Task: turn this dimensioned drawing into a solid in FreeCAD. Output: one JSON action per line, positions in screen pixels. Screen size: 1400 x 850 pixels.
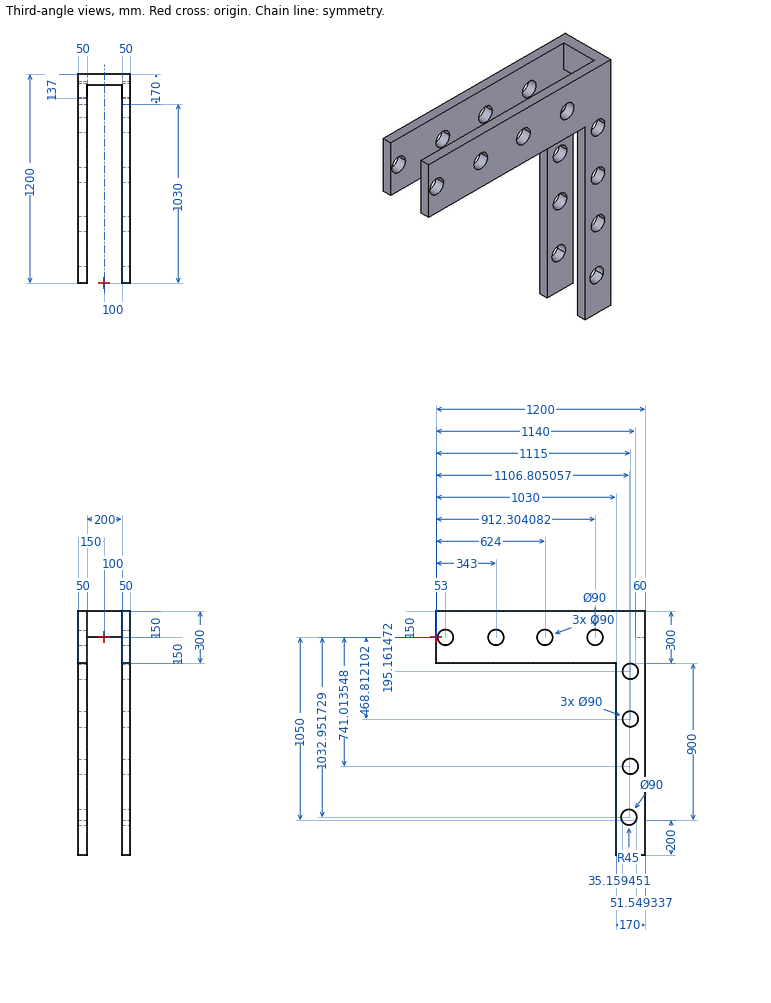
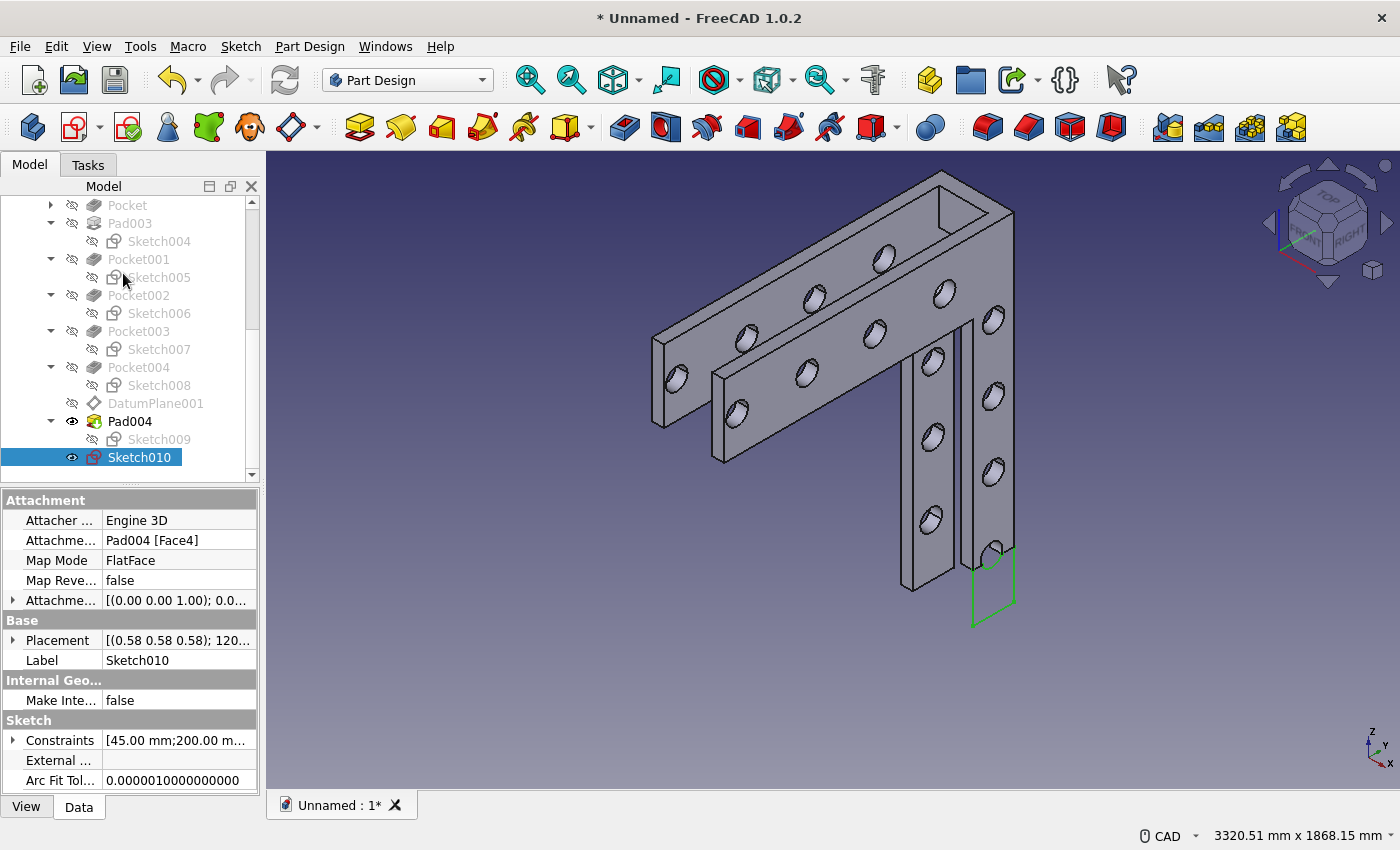
{"action": "left_click", "coordinate": [360, 128]}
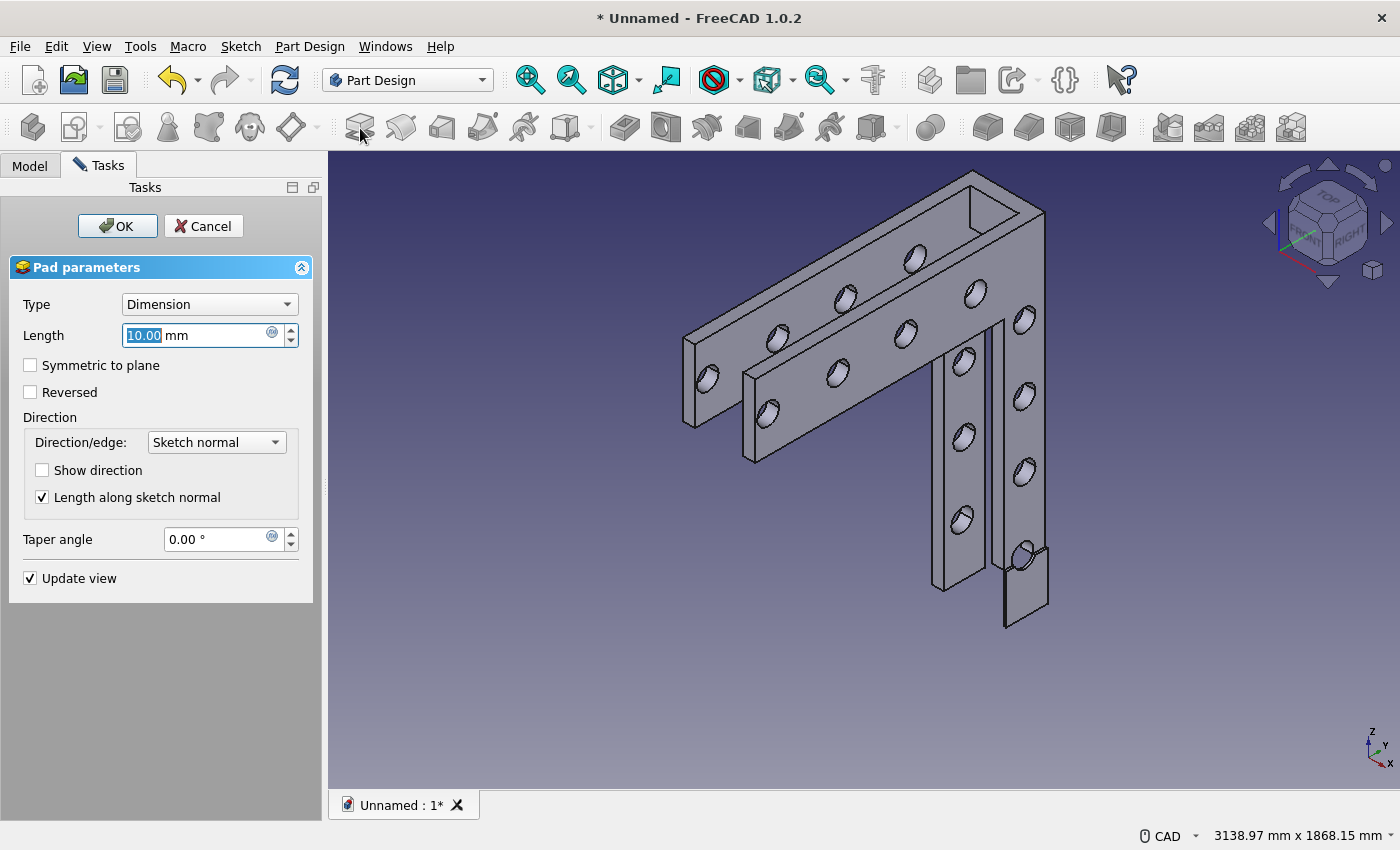
{"action": "type", "text": "50"}
{"action": "key", "text": "Tab"}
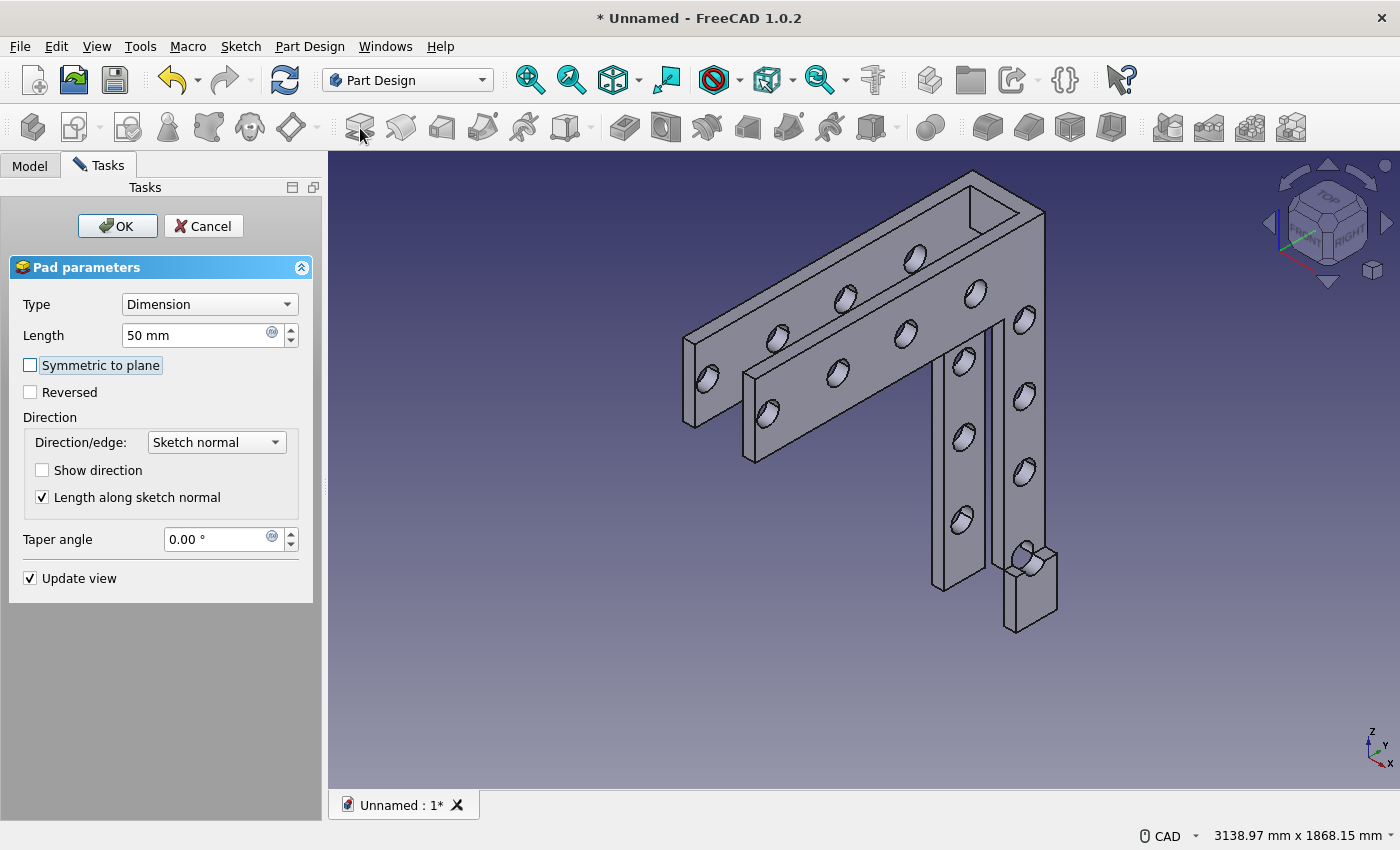
{"action": "left_click", "coordinate": [31, 392]}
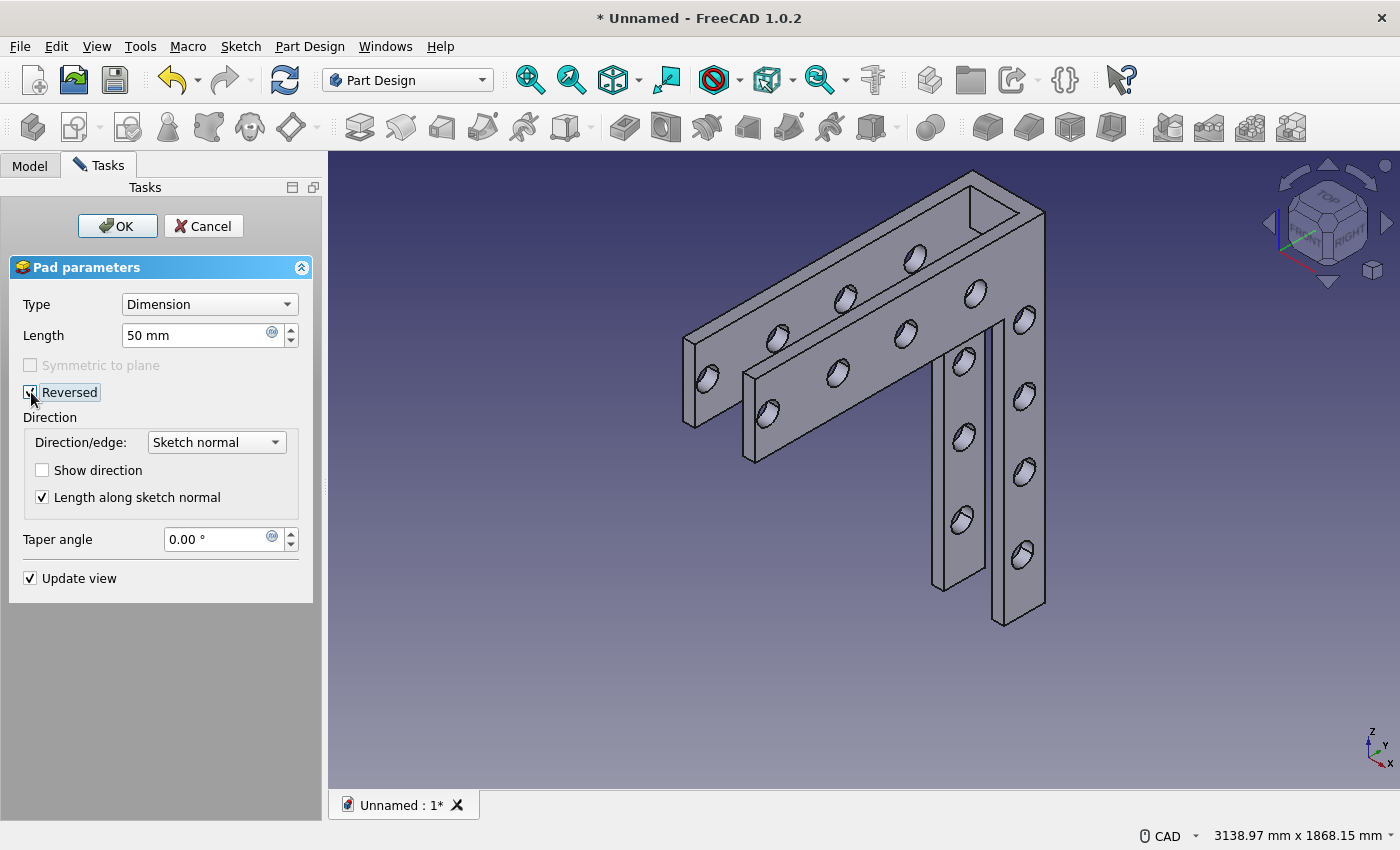
{"action": "left_click", "coordinate": [118, 226]}